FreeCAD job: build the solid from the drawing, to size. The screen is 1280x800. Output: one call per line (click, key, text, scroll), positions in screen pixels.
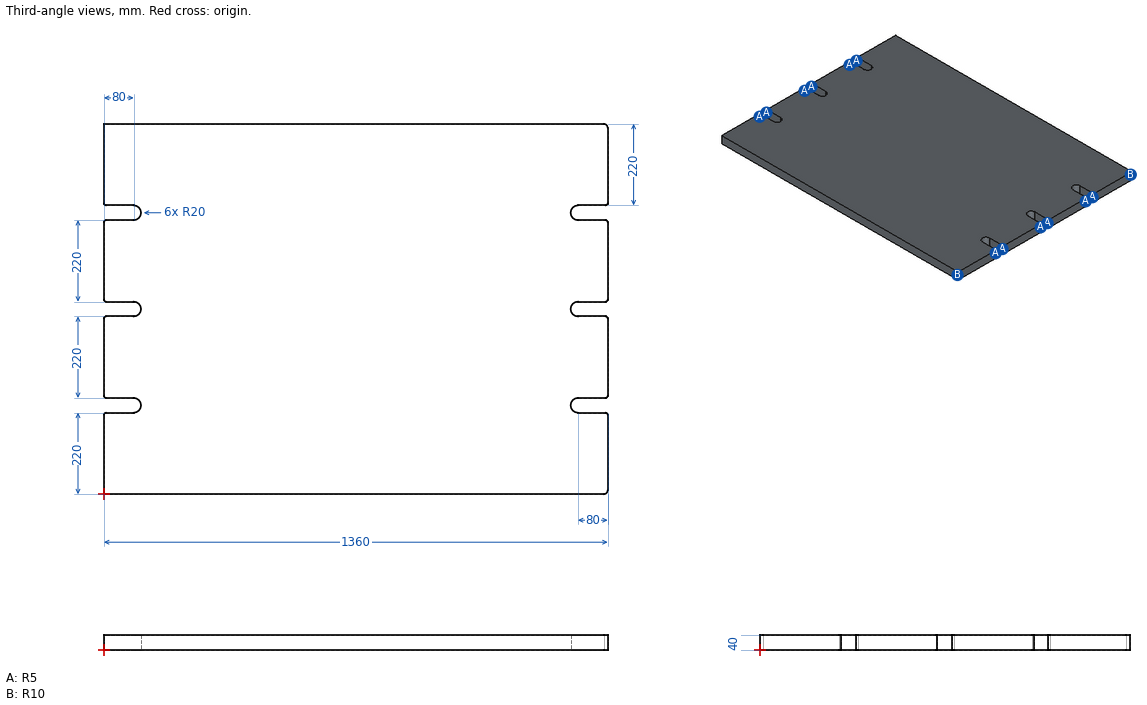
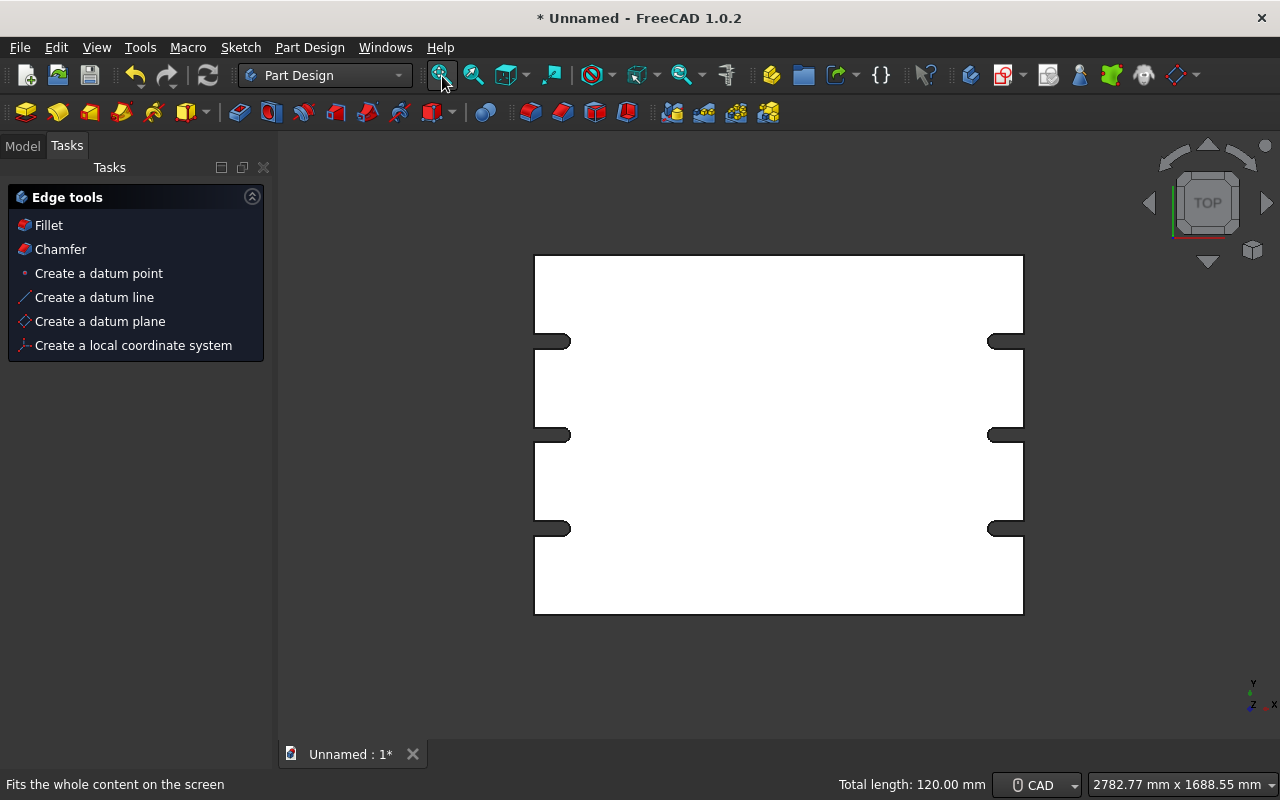
scroll(534, 535, up, 6)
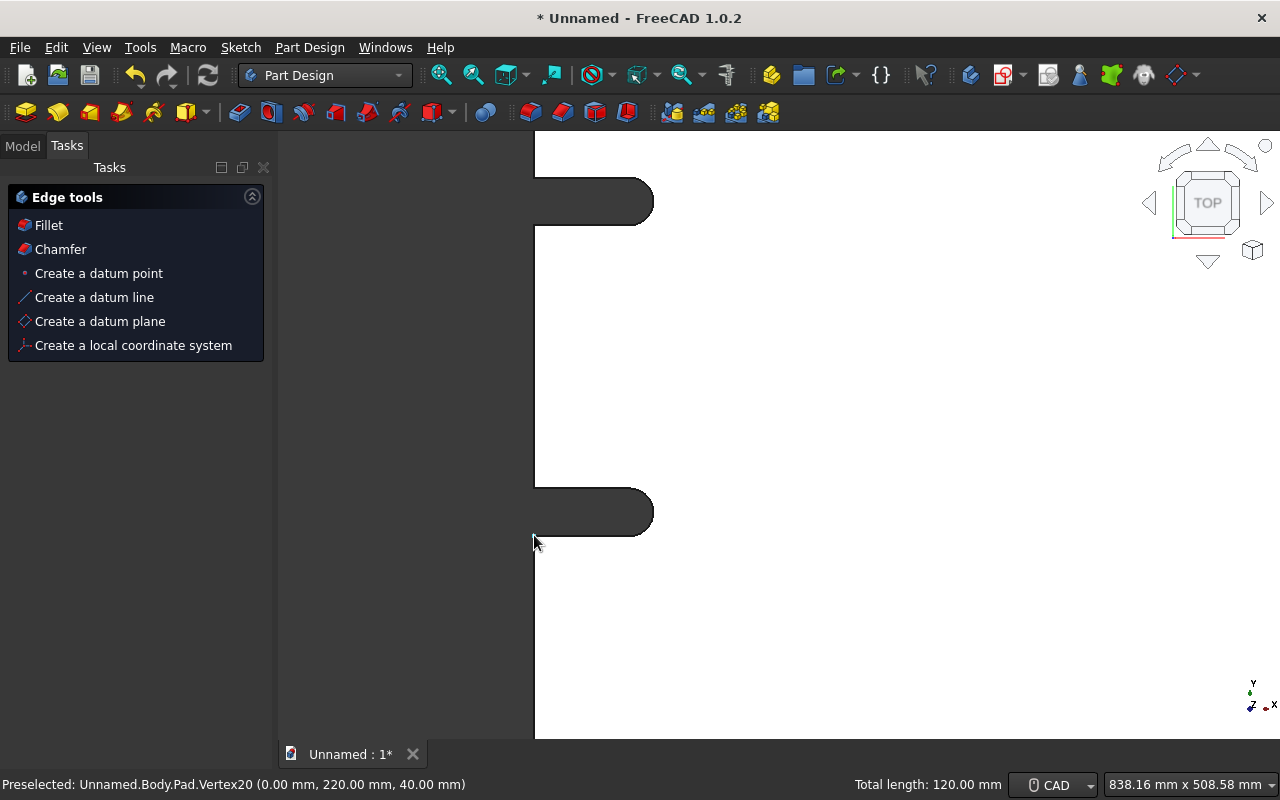
click(442, 76)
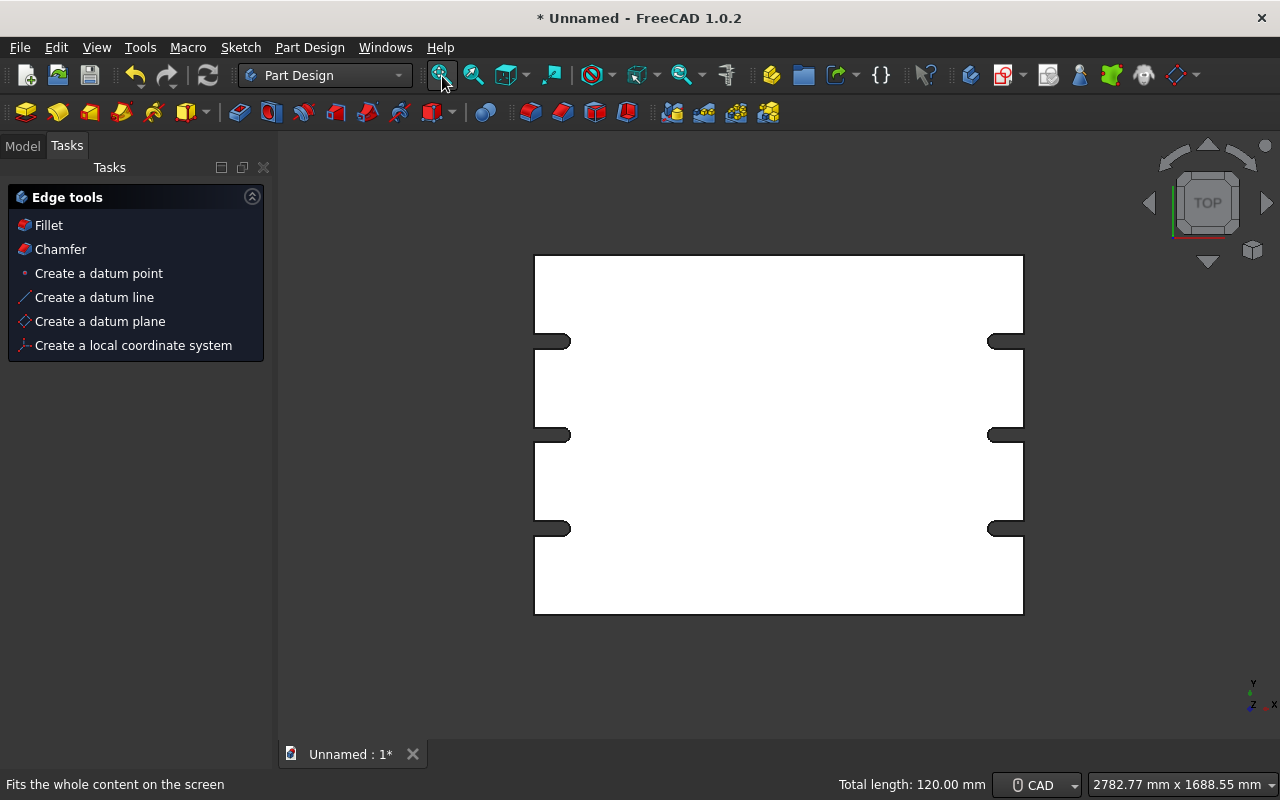
key(1)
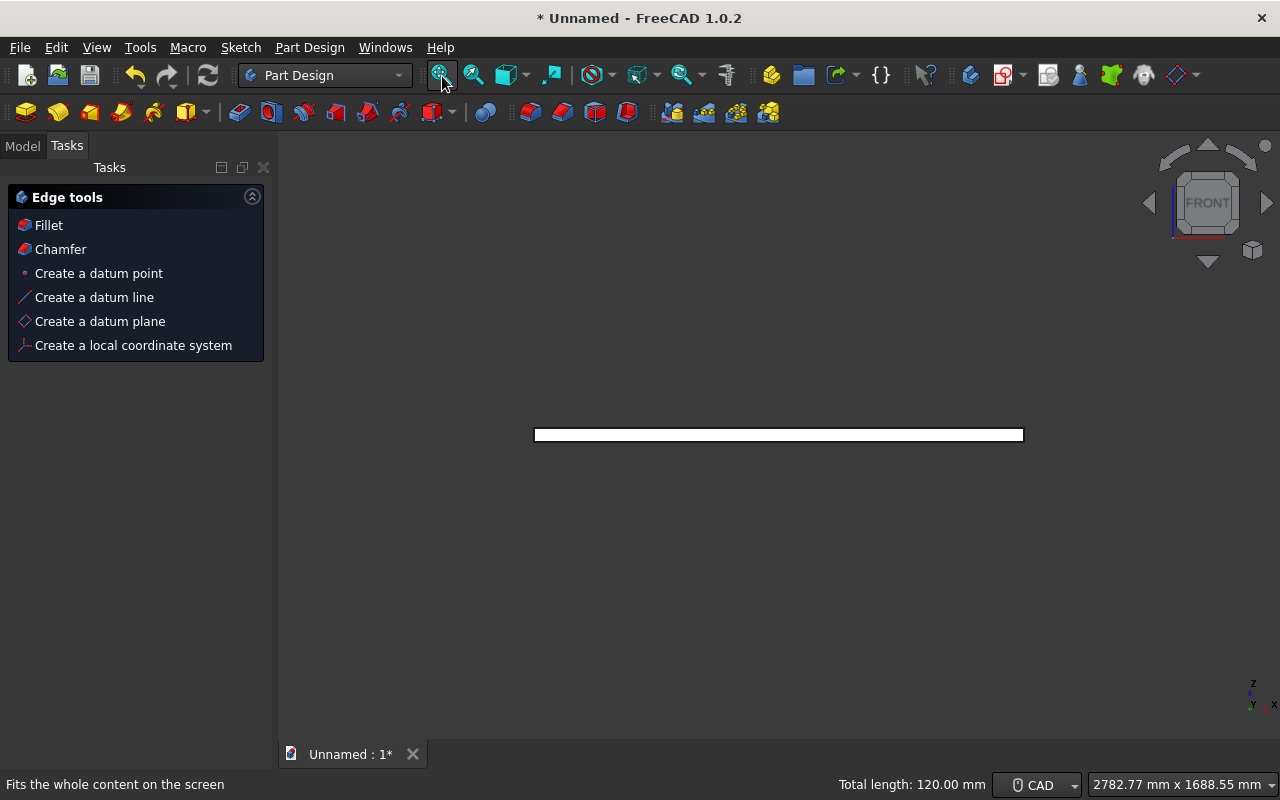
scroll(534, 434, up, 6)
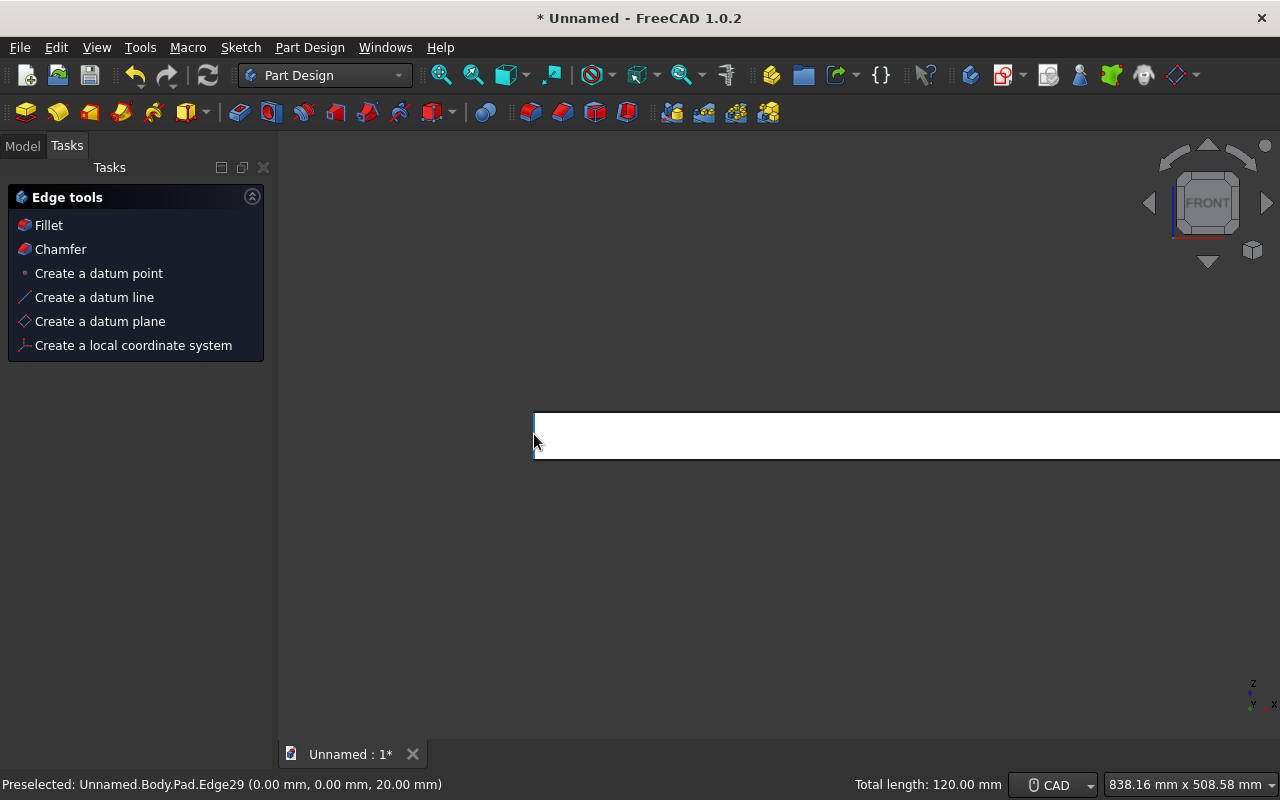
click(442, 76)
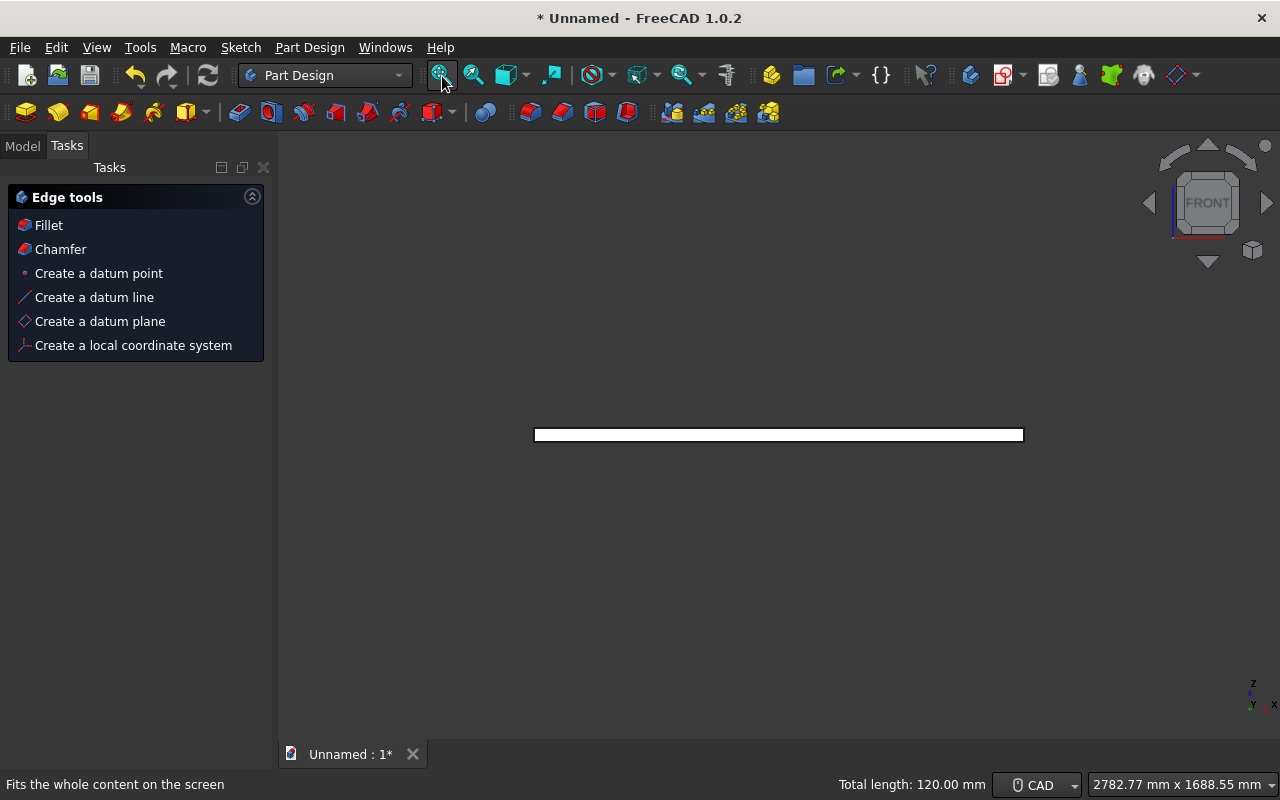
key(3)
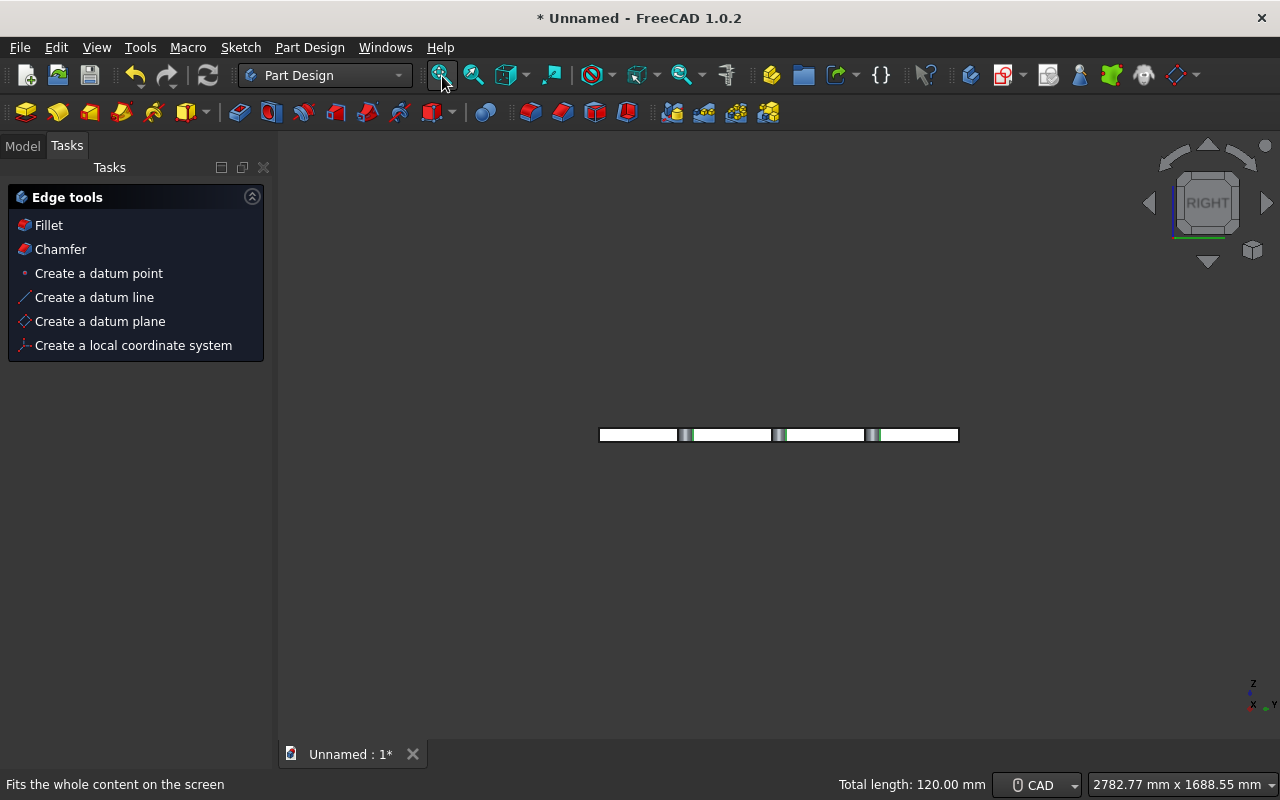
click(442, 76)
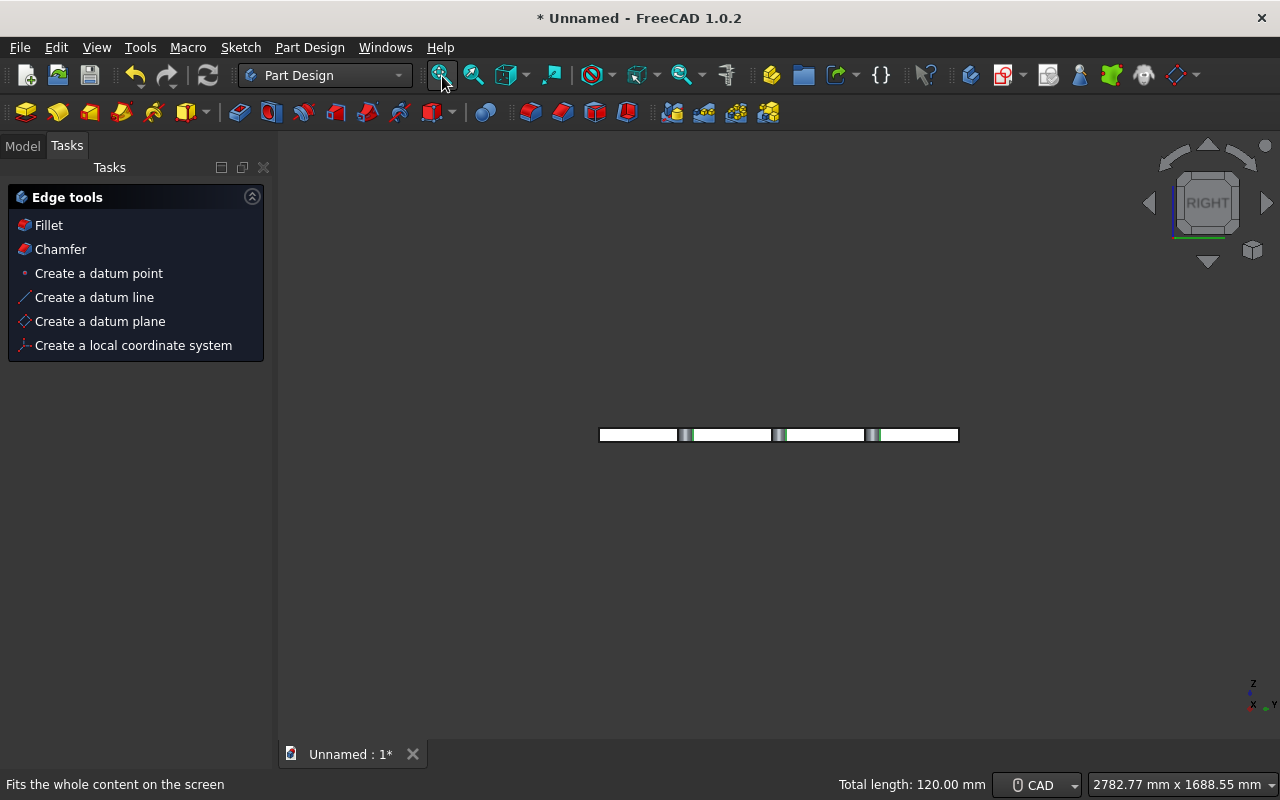
click(865, 434, ctrl)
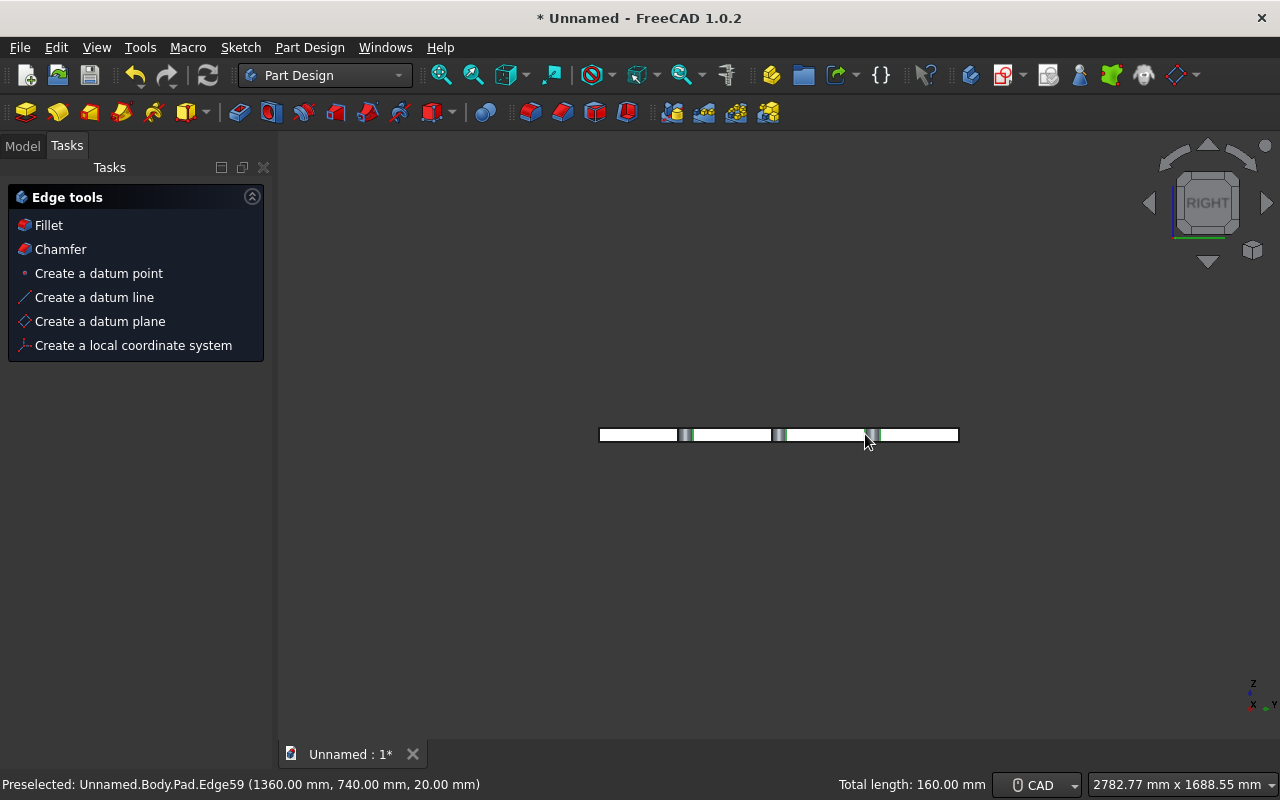
click(772, 434, ctrl)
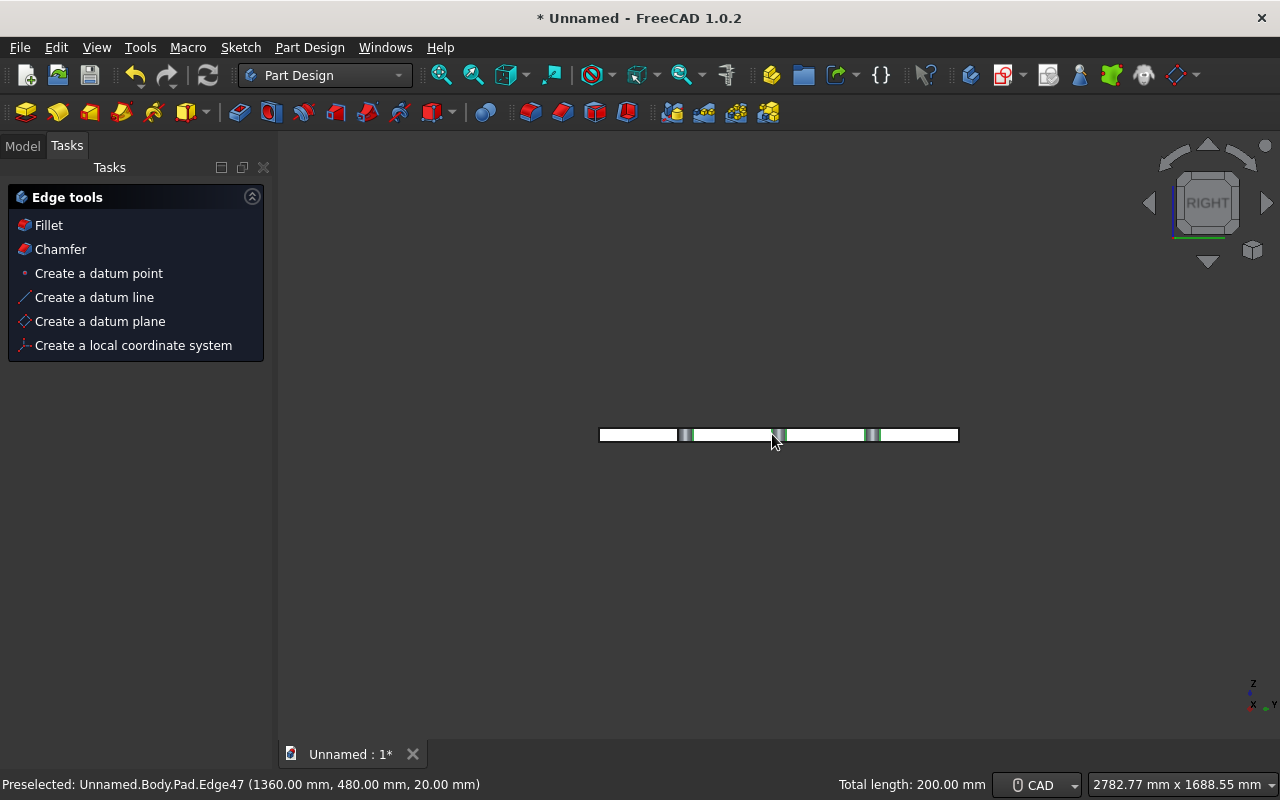
click(678, 434, ctrl)